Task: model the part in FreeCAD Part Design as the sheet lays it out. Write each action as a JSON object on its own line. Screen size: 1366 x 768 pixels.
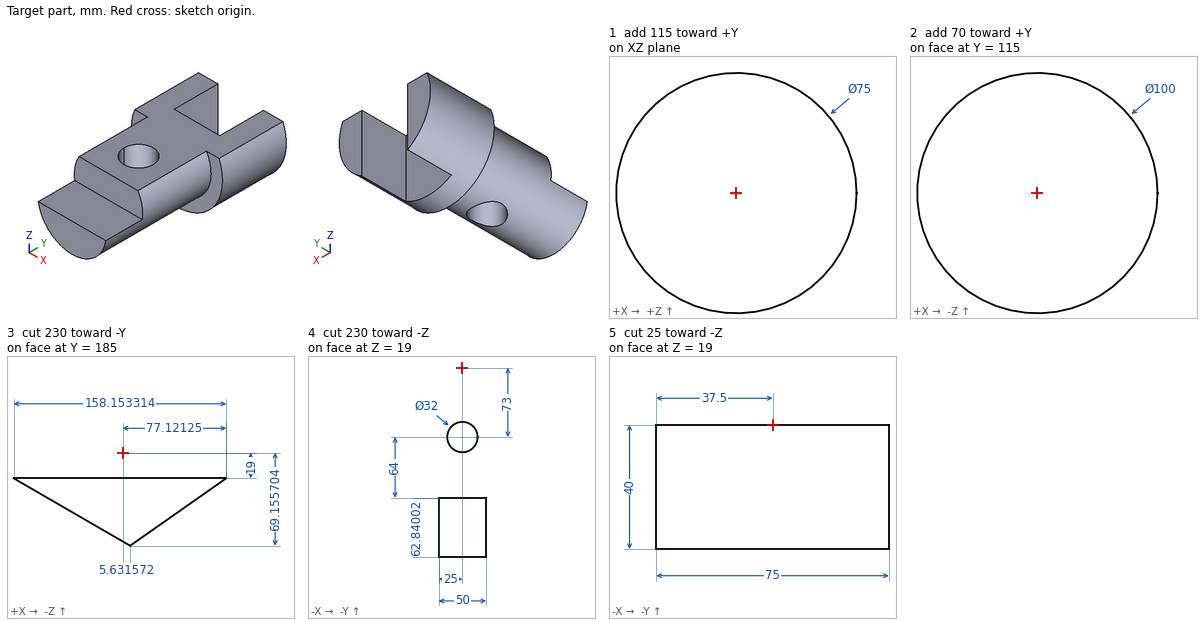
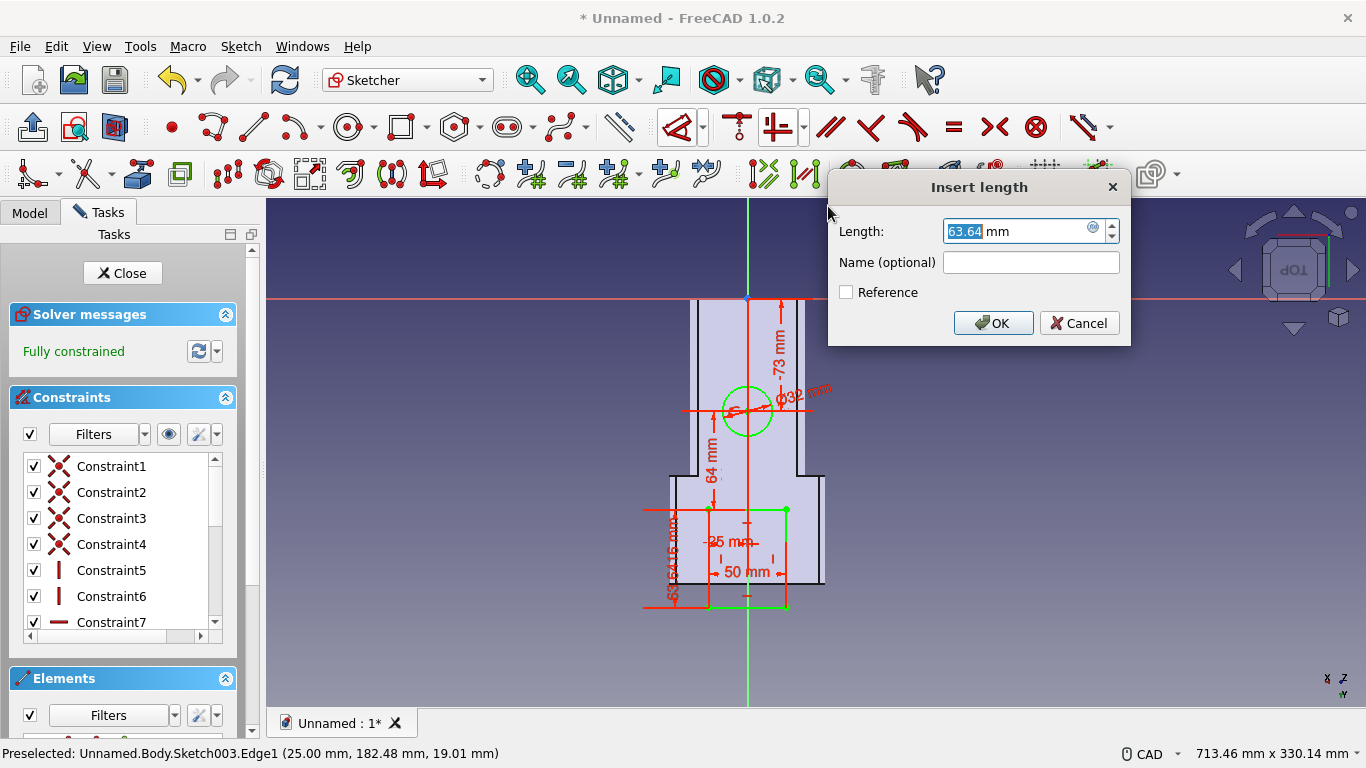
{"action": "type", "text": "62.84002"}
{"action": "key", "text": "Return"}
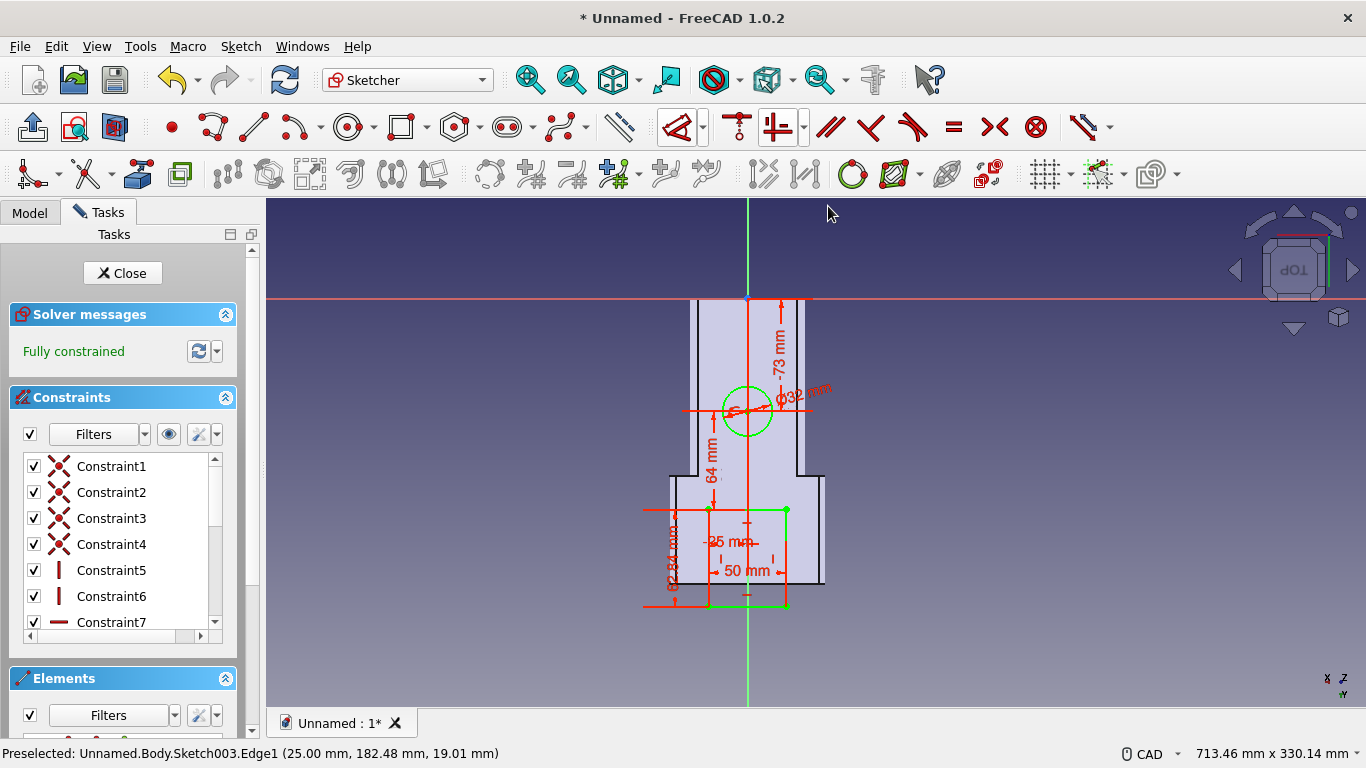
{"action": "left_click", "coordinate": [123, 273]}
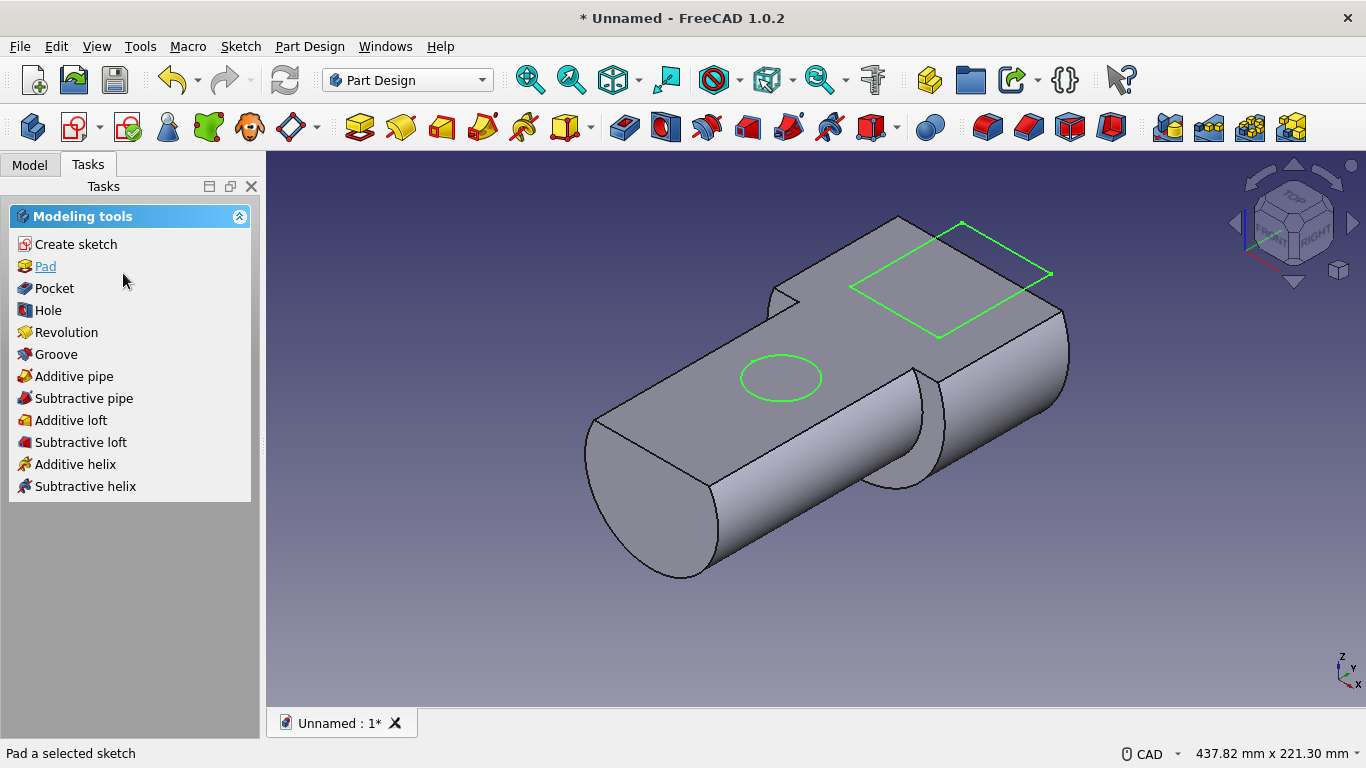
{"action": "left_click", "coordinate": [625, 128]}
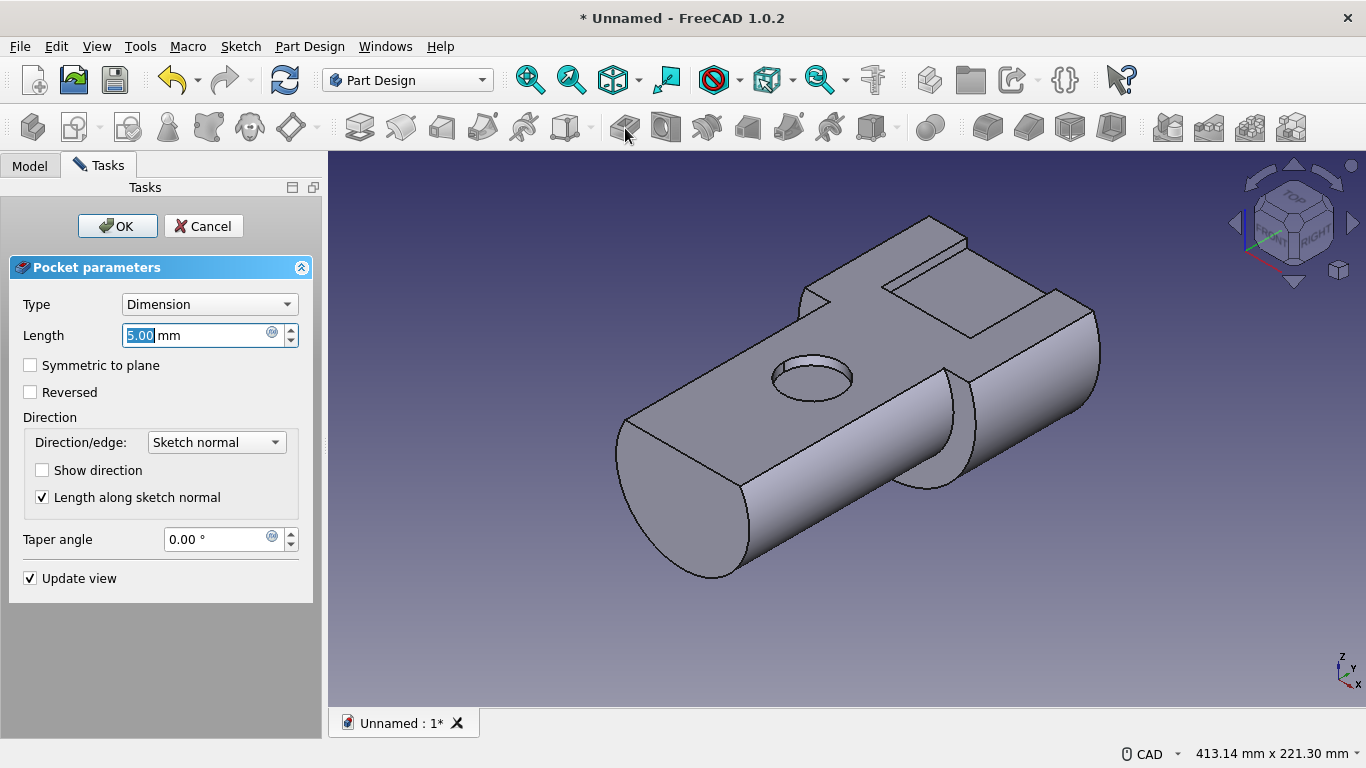
{"action": "type", "text": "230"}
{"action": "key", "text": "Tab"}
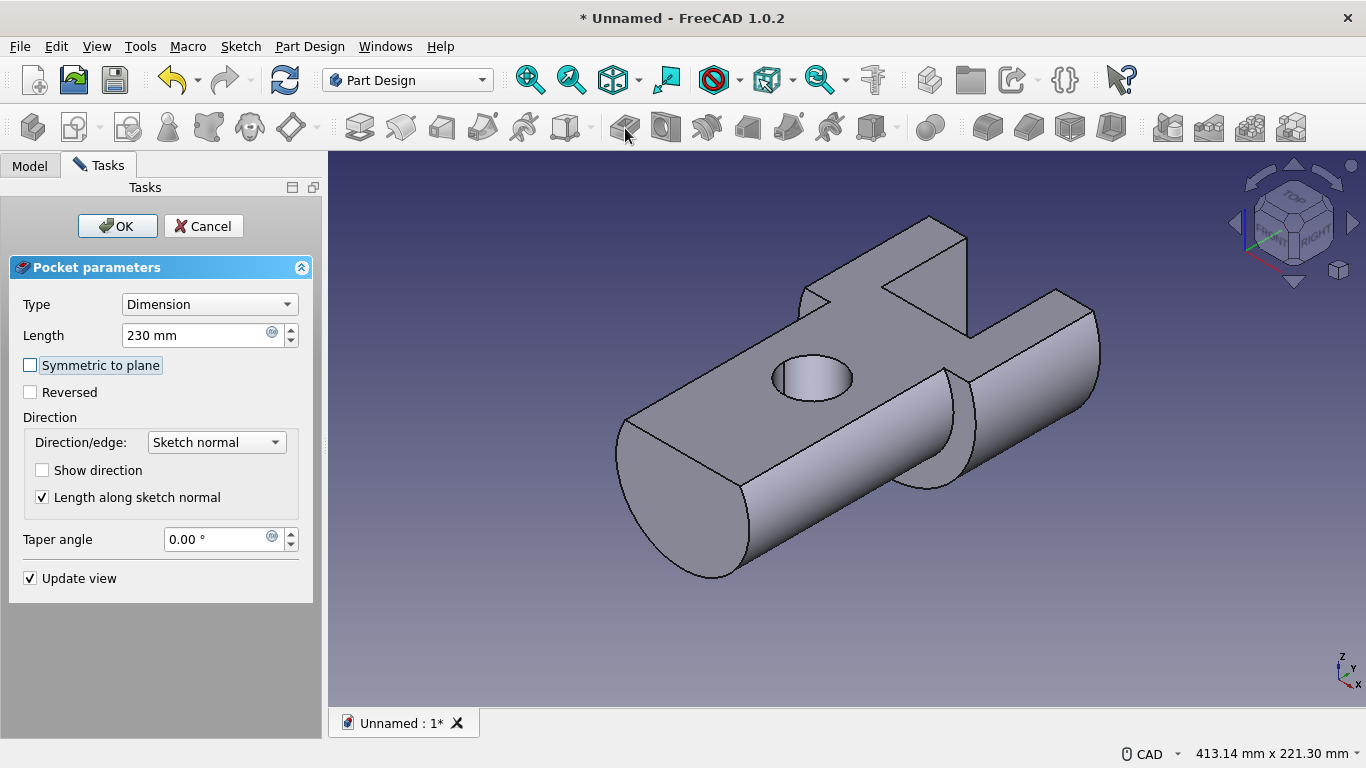
{"action": "left_click", "coordinate": [118, 226]}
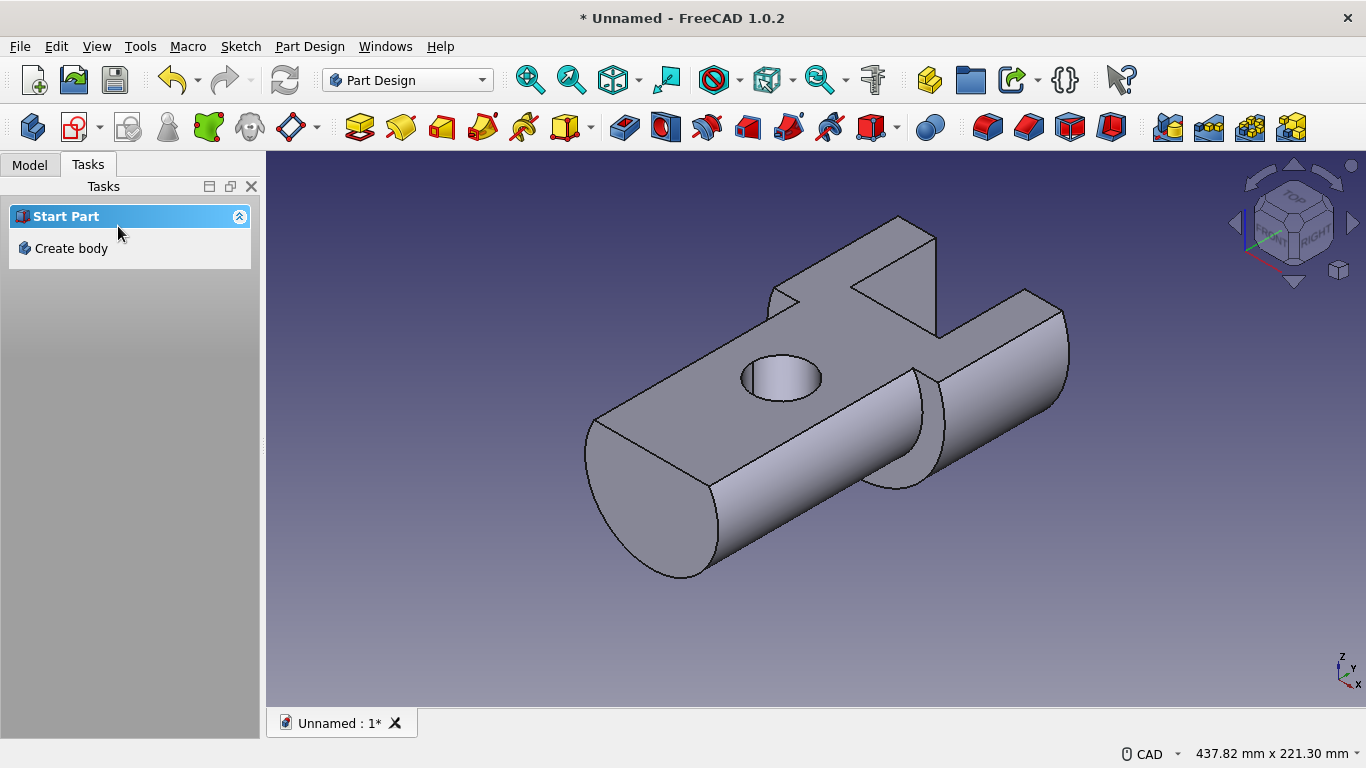
{"action": "left_click", "coordinate": [746, 425]}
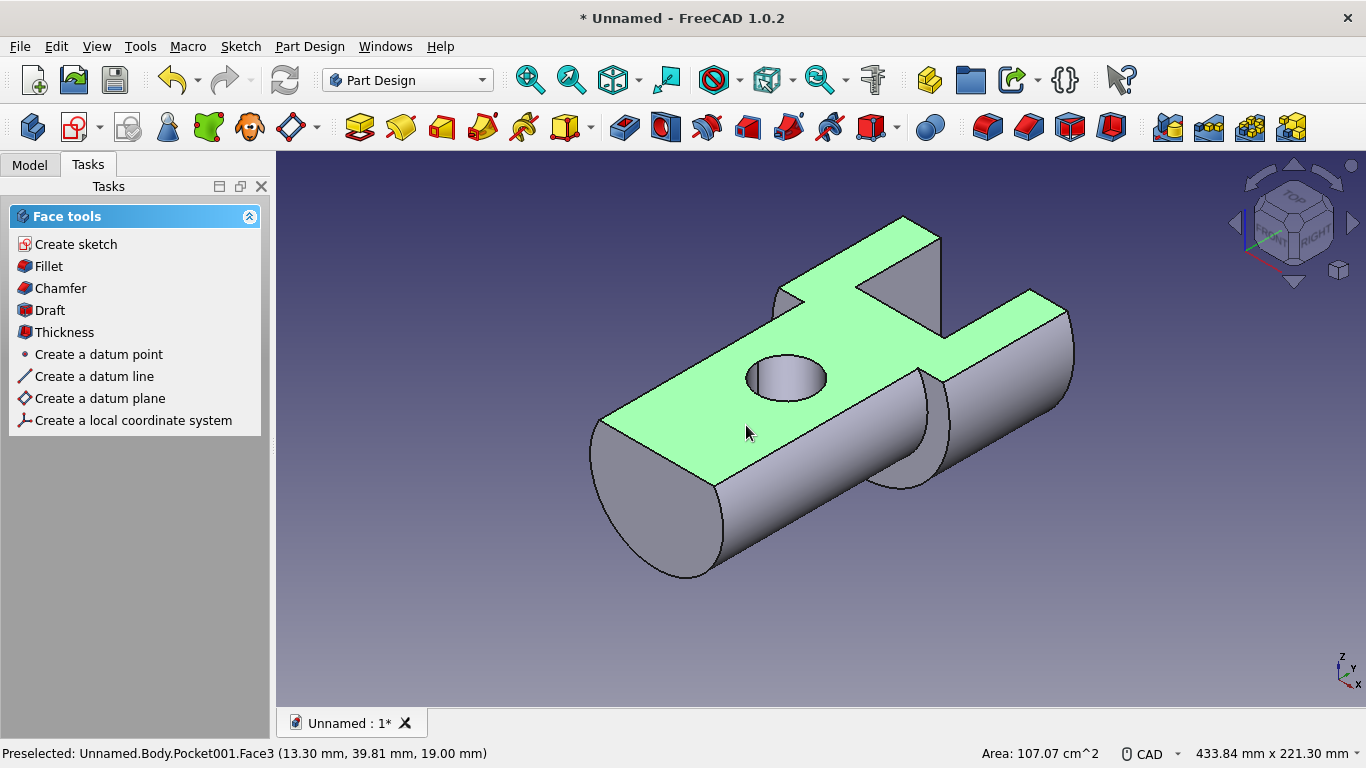
{"action": "left_click", "coordinate": [74, 128]}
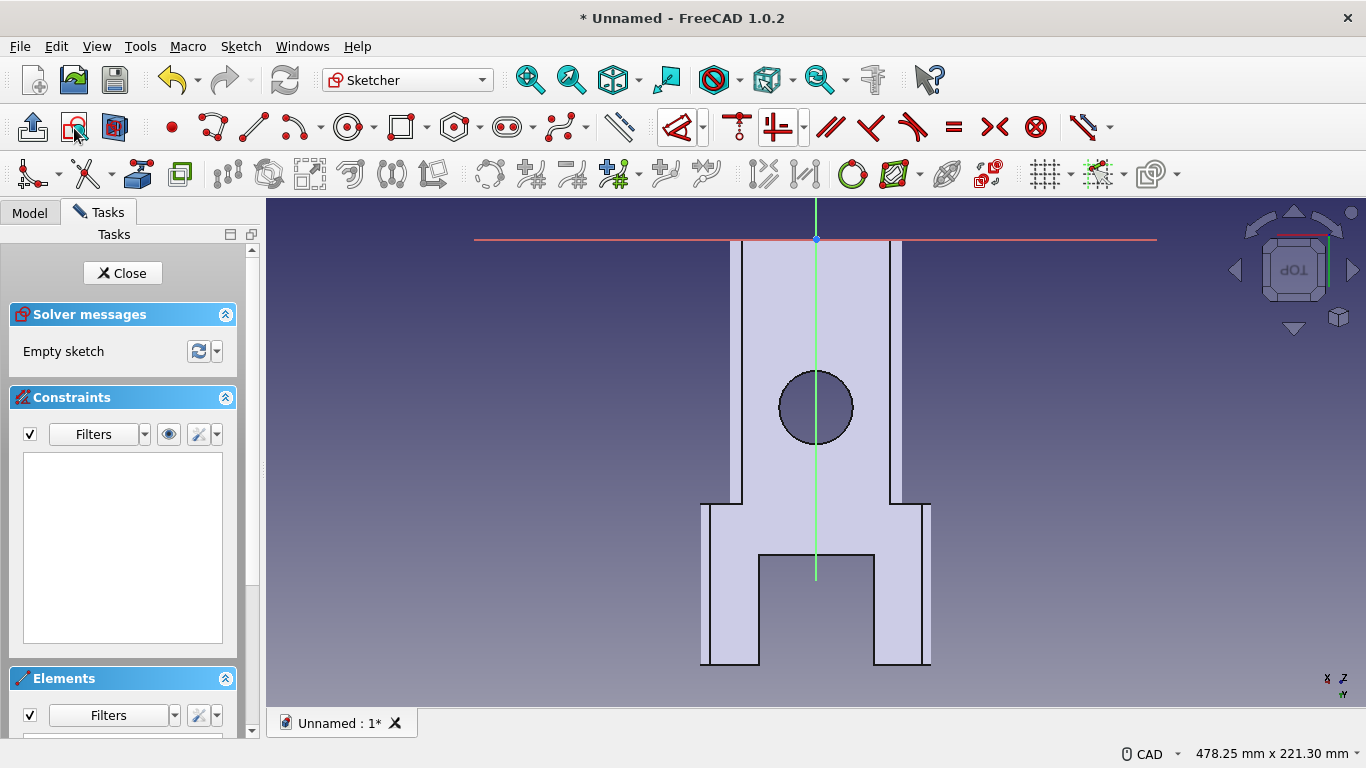
{"action": "scroll", "coordinate": [846, 226], "scroll_direction": "up", "scroll_amount": 6}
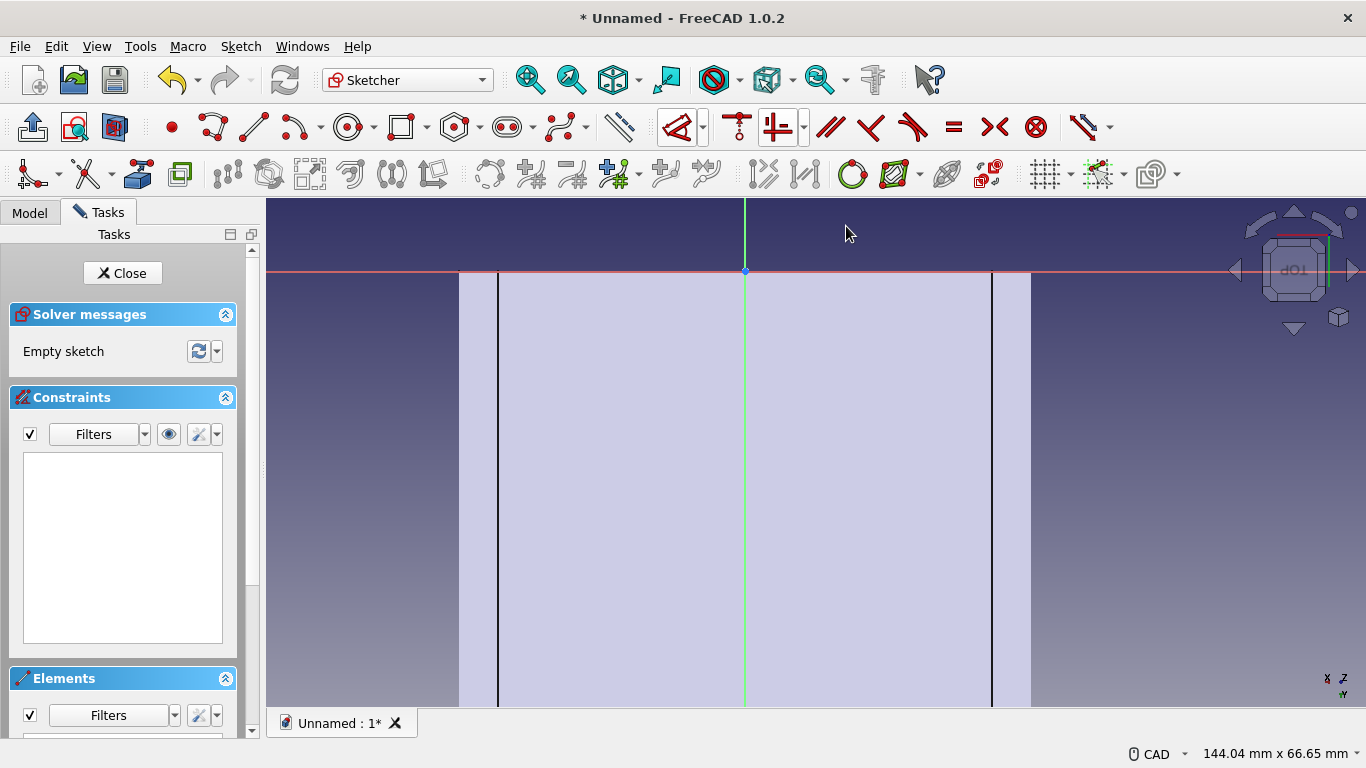
{"action": "left_click", "coordinate": [400, 128]}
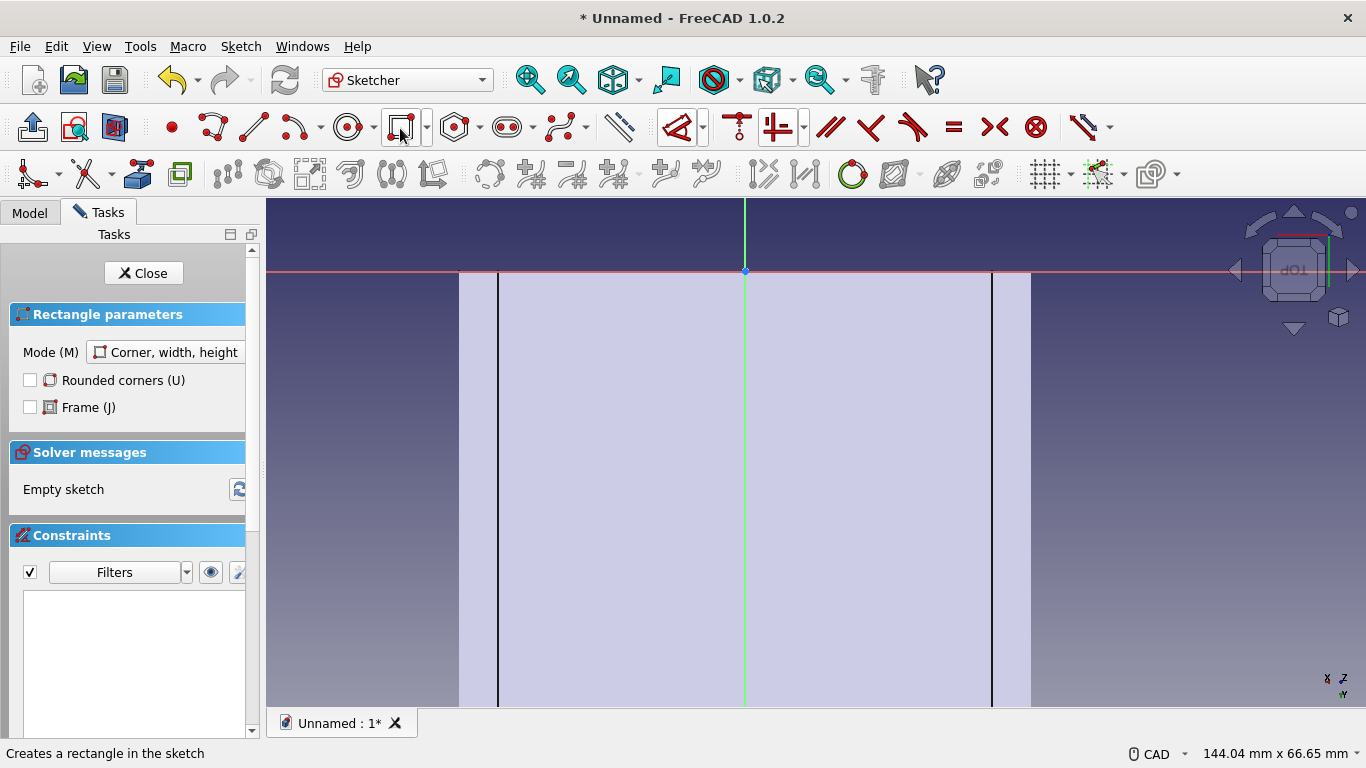
{"action": "left_click", "coordinate": [459, 272]}
{"action": "left_click", "coordinate": [1032, 577]}
{"action": "key", "text": "Escape"}